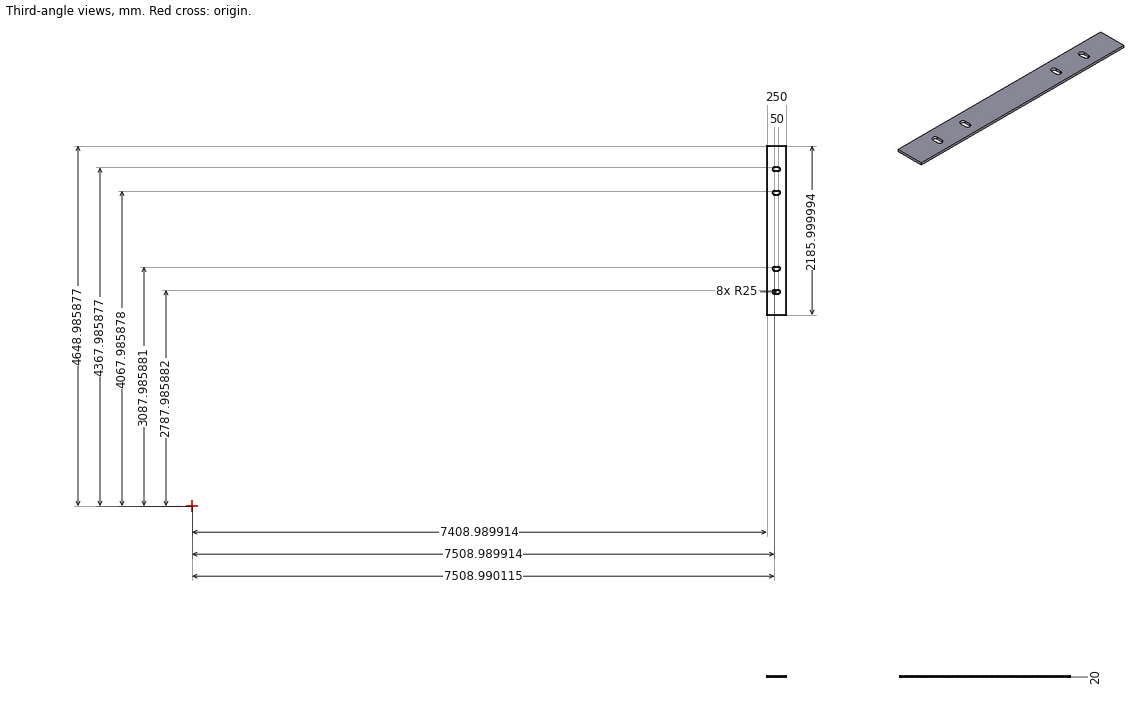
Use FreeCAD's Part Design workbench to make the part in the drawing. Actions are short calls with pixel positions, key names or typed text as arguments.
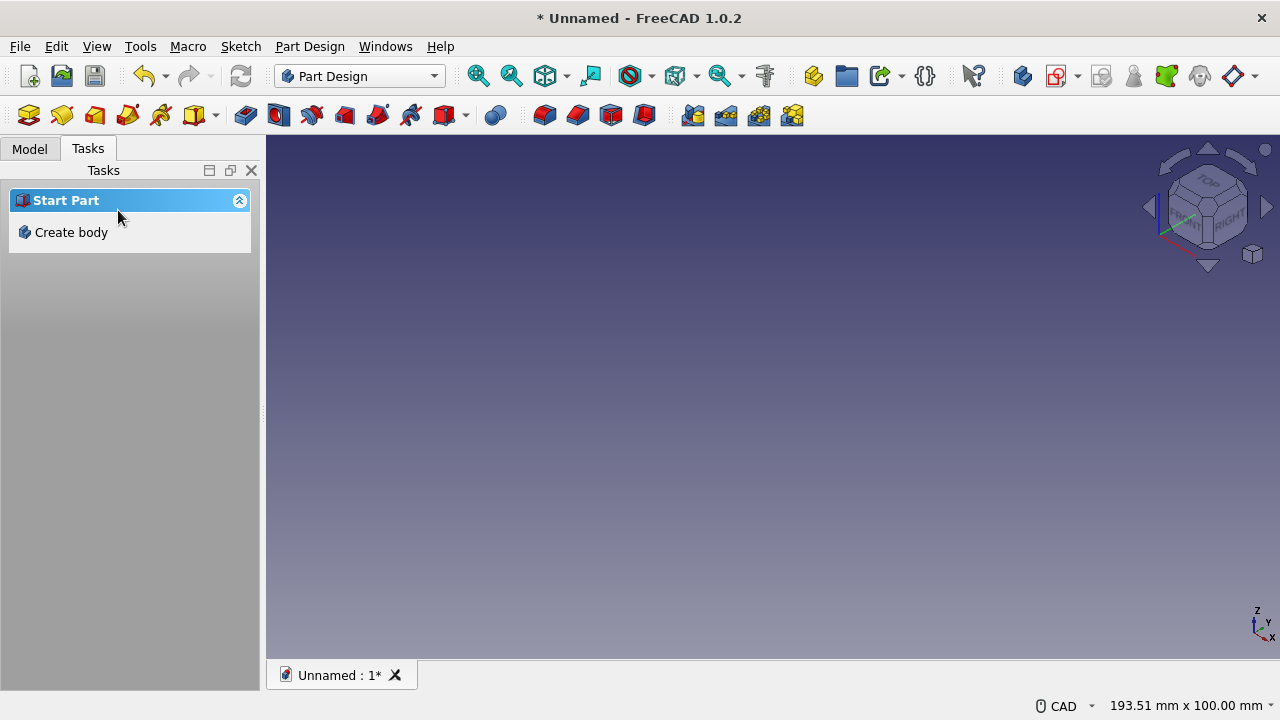
key(v)
key(f)